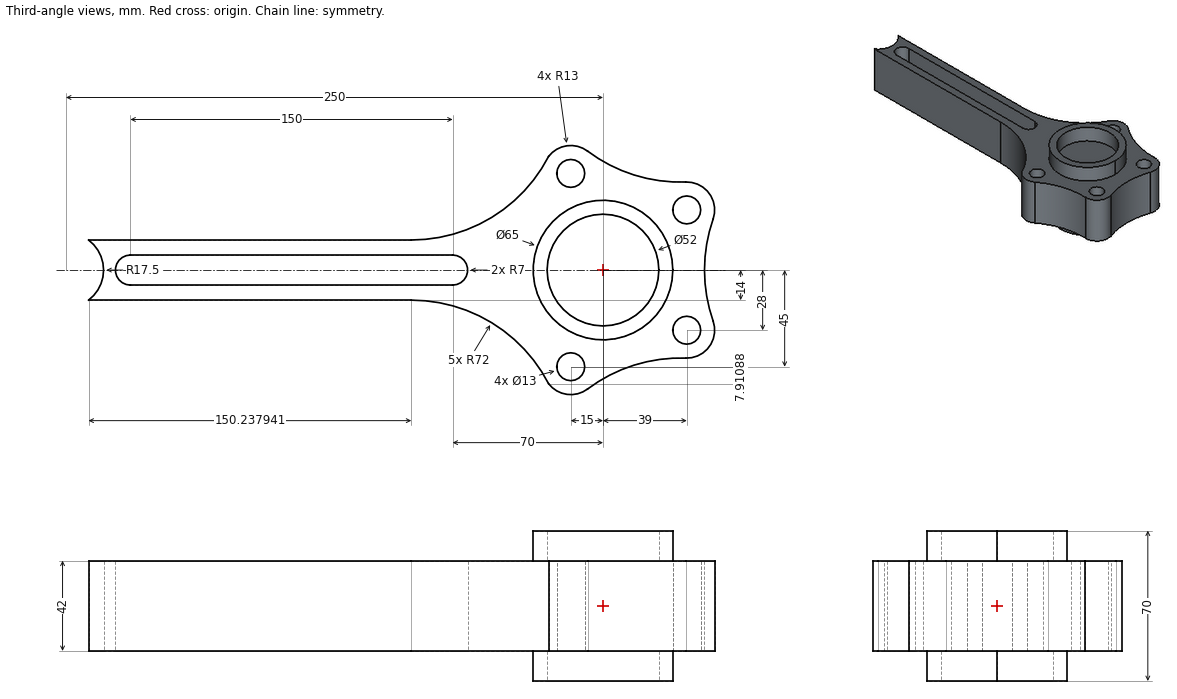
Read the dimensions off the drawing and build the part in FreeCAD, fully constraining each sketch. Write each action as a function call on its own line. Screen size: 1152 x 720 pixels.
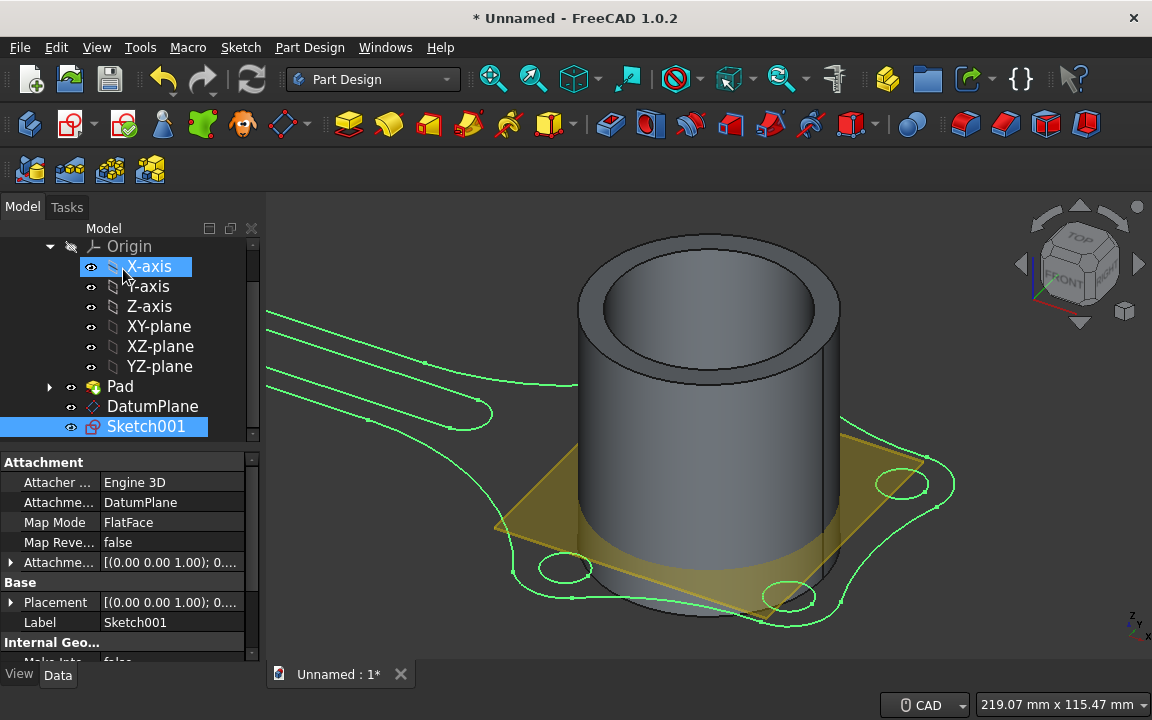
click(350, 124)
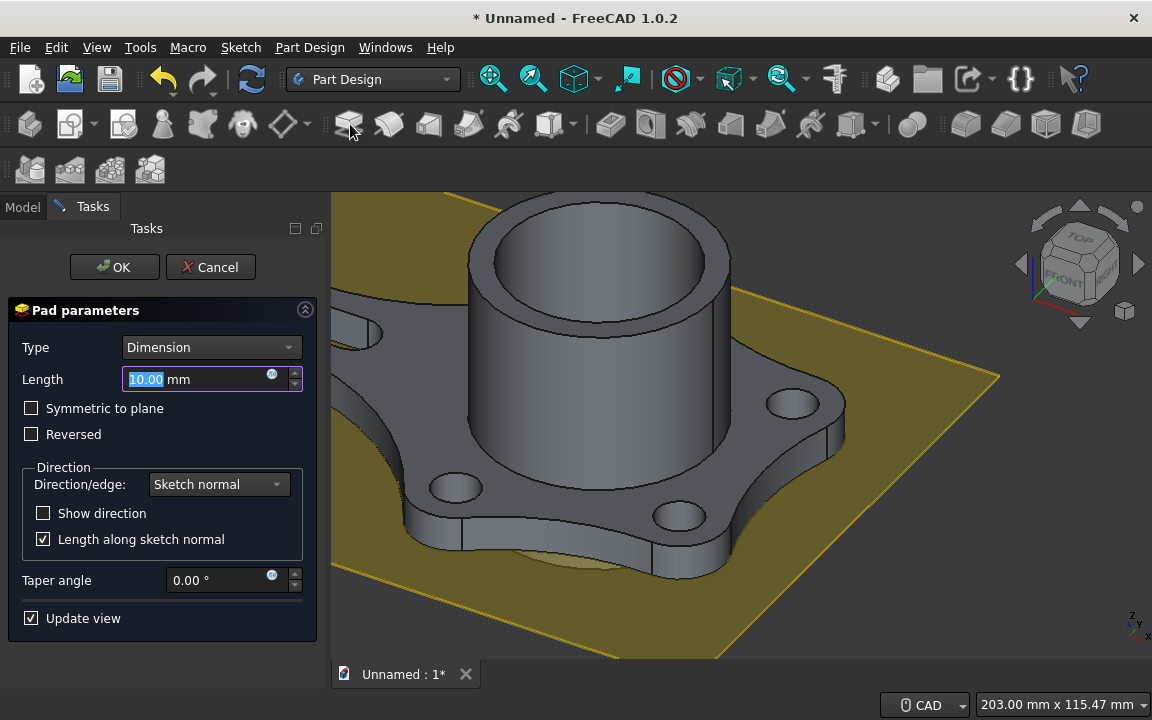
text(42)
key(Tab)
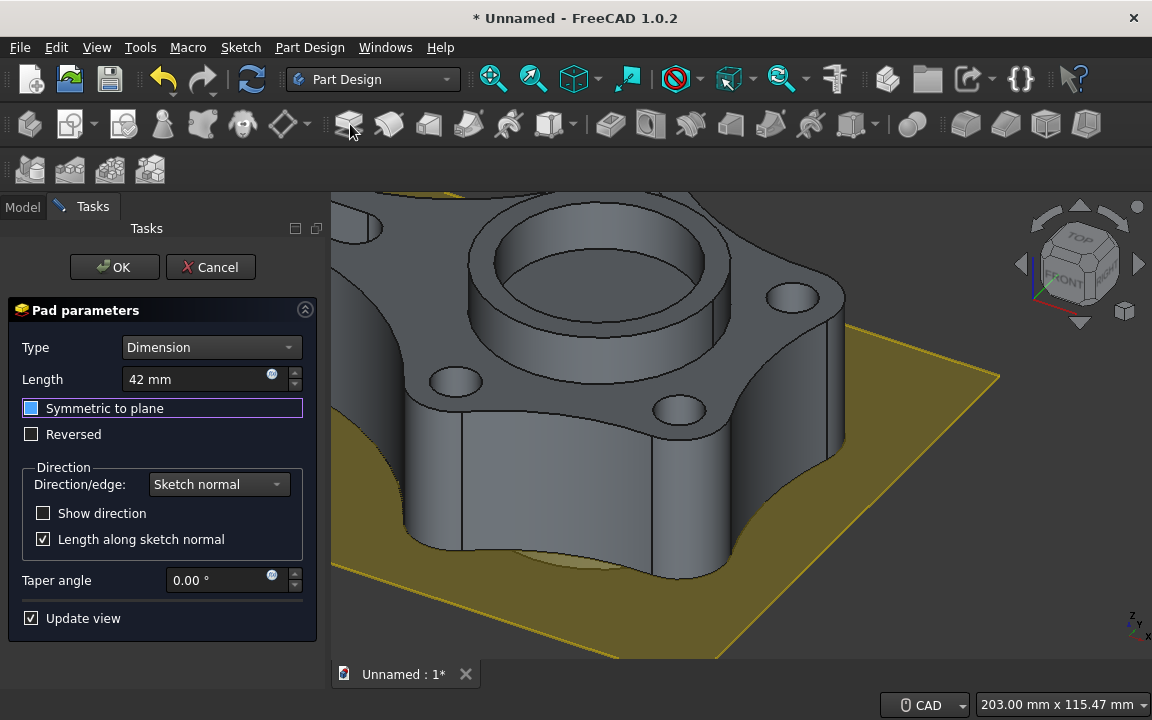
click(115, 267)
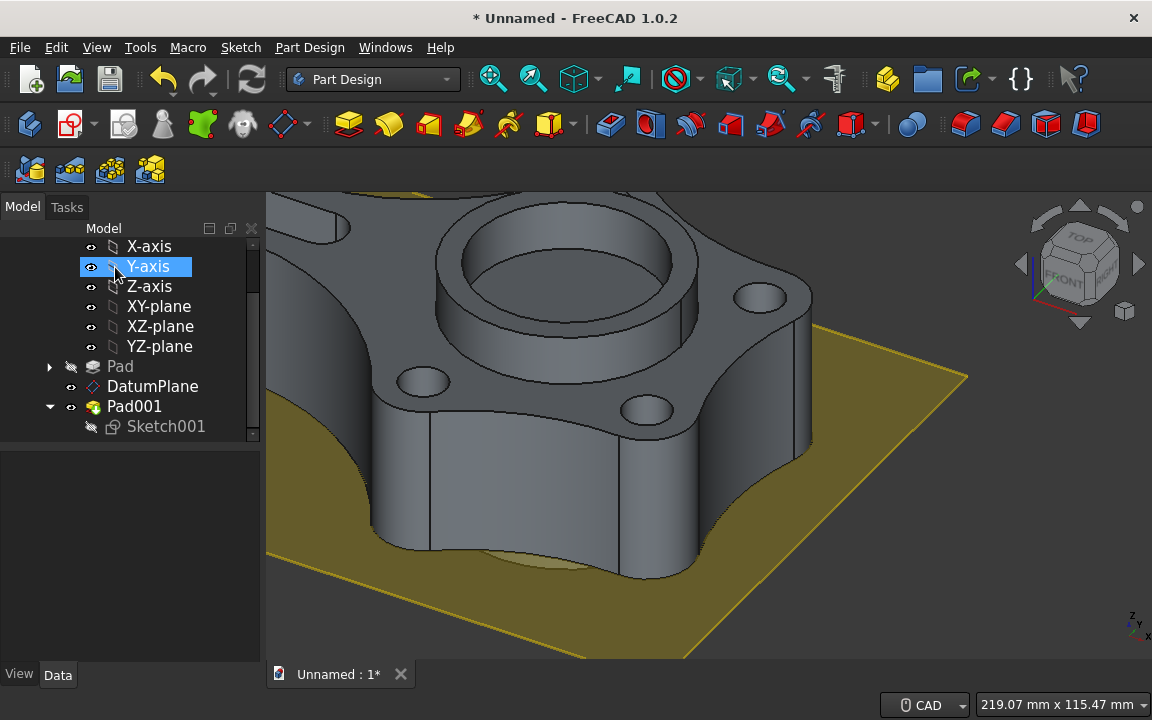
click(116, 387)
key(space)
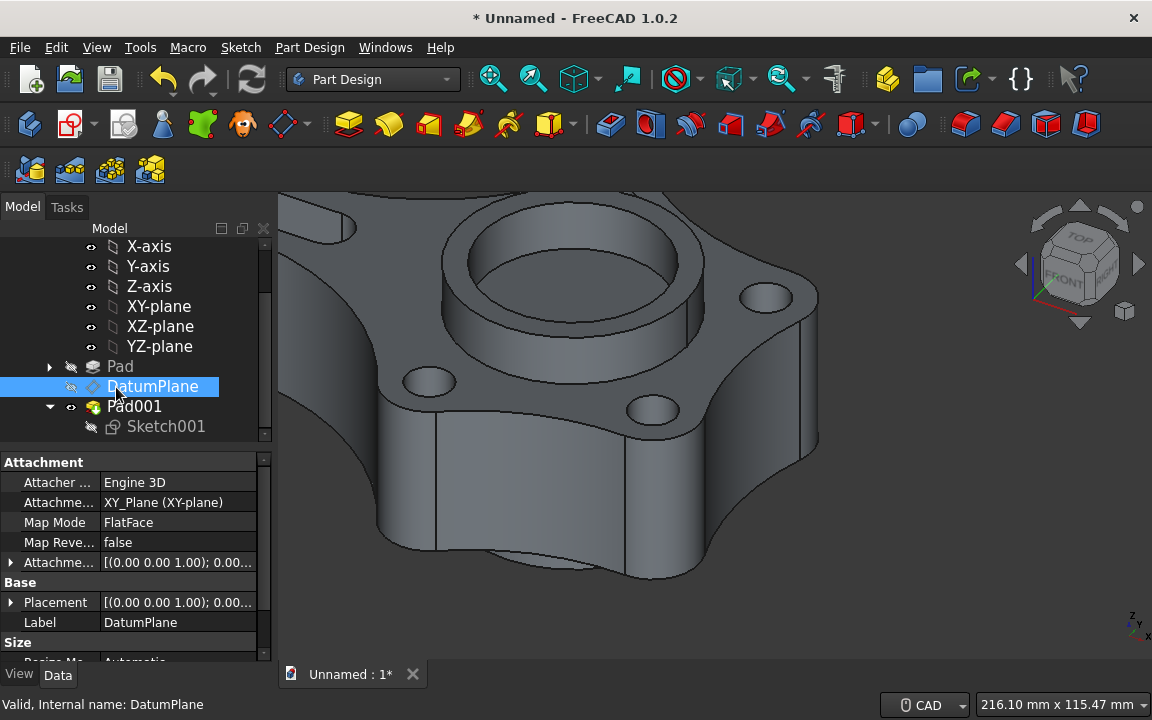
key(0)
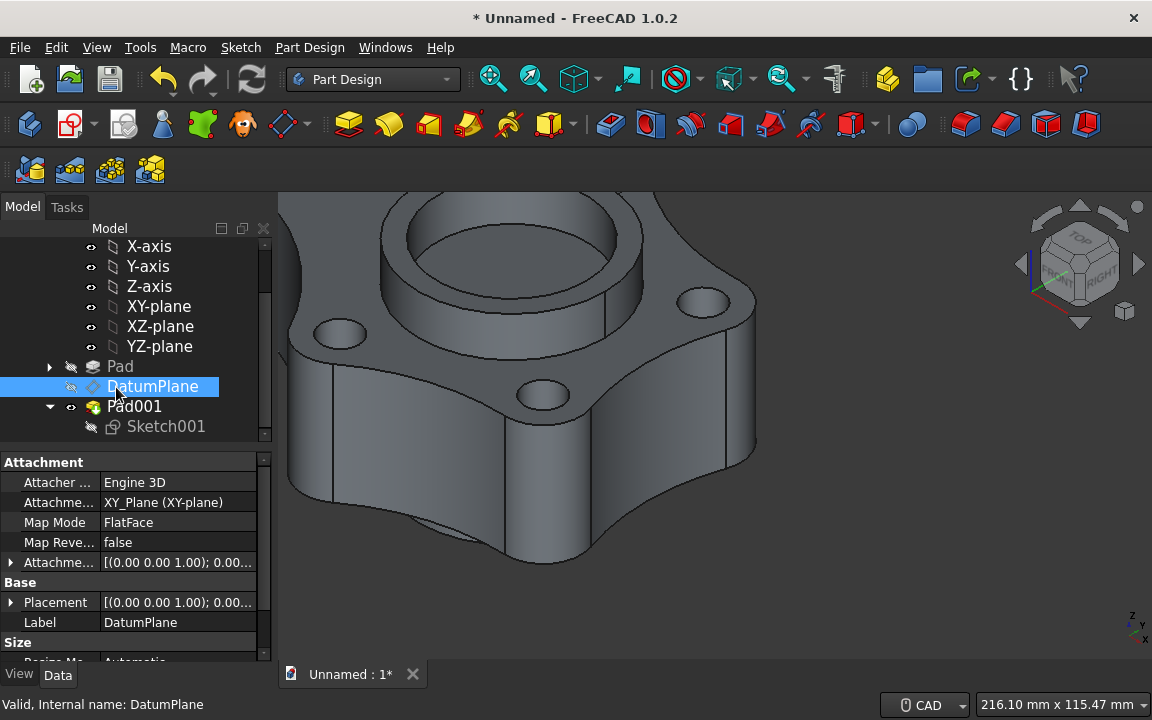
click(494, 80)